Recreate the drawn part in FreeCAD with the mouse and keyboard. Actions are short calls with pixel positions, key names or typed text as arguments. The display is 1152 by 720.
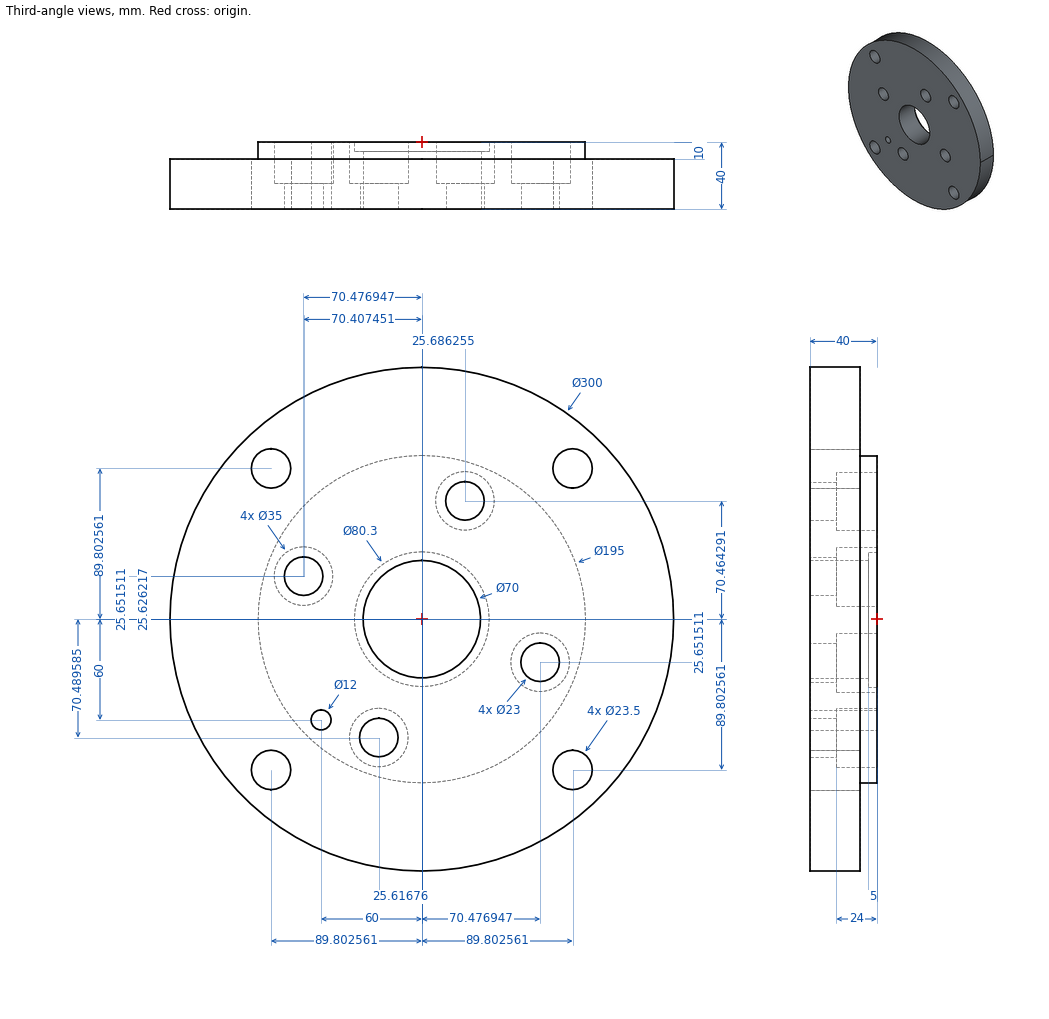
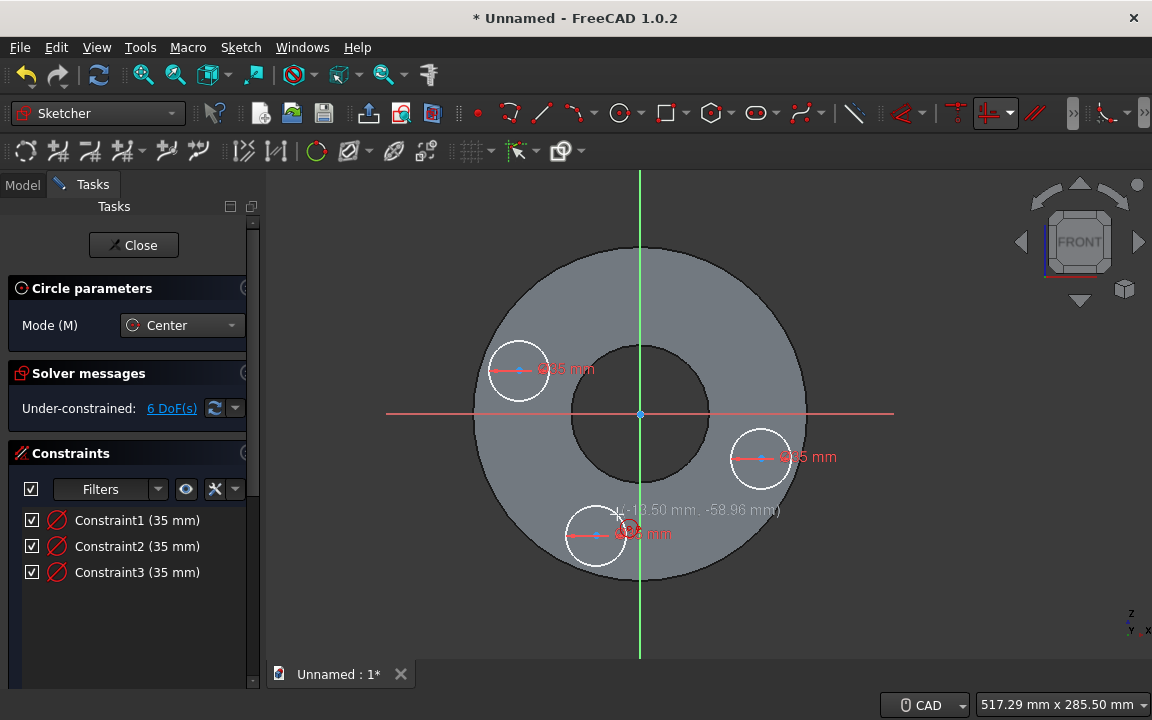
click(684, 293)
move(705, 272)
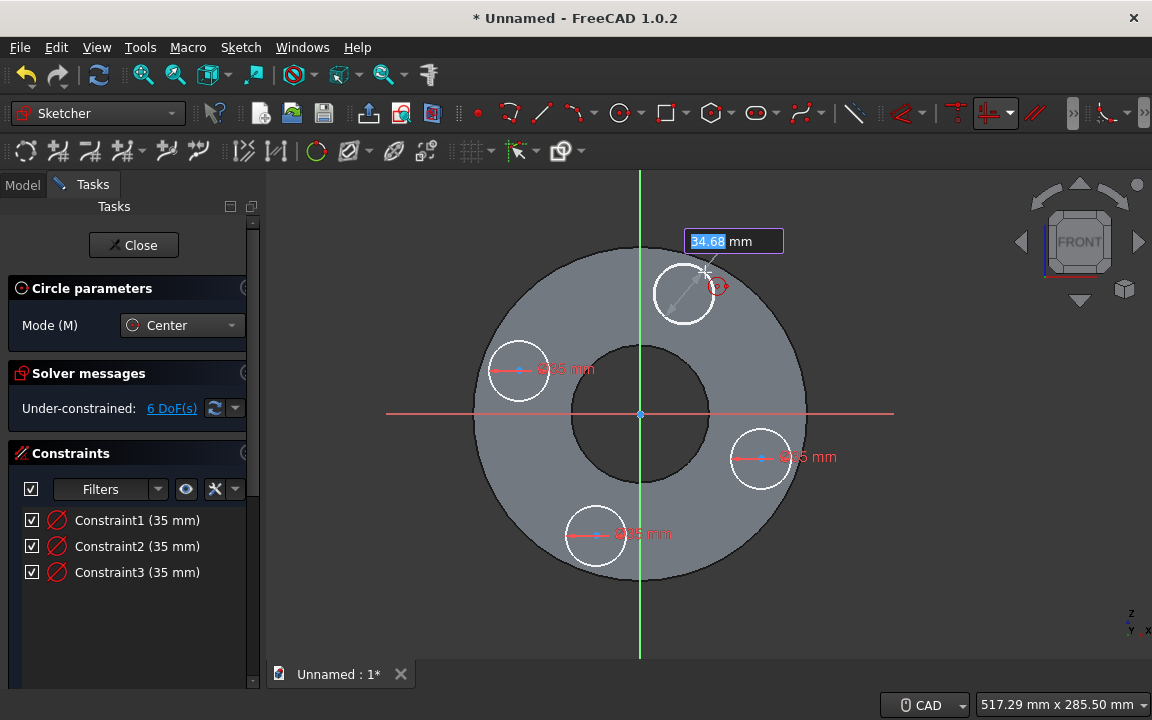
text(35)
key(Return)
key(Escape)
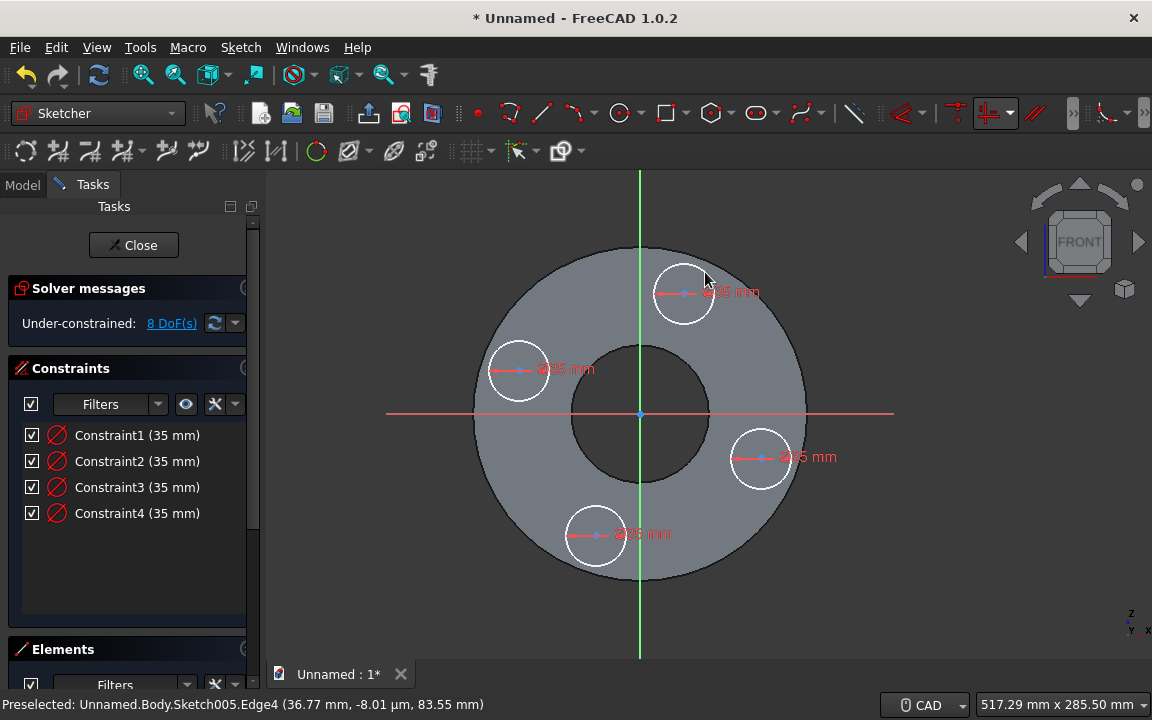
click(902, 114)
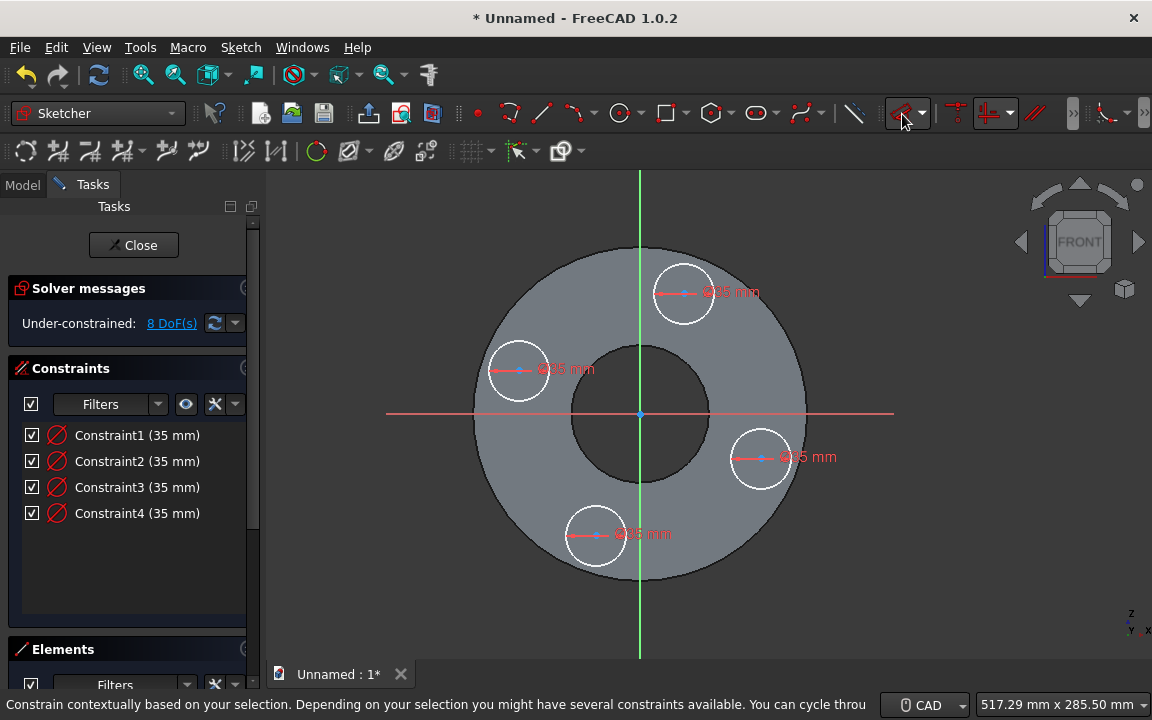
click(596, 536)
click(618, 380)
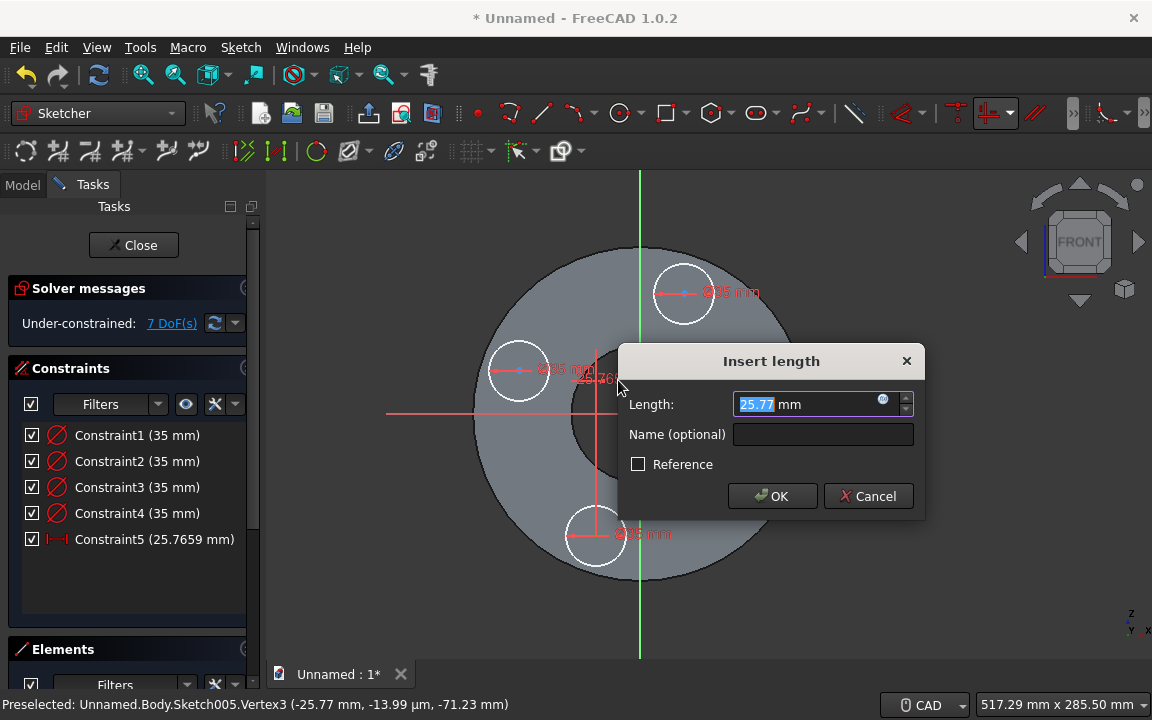
text(25.61676)
key(Return)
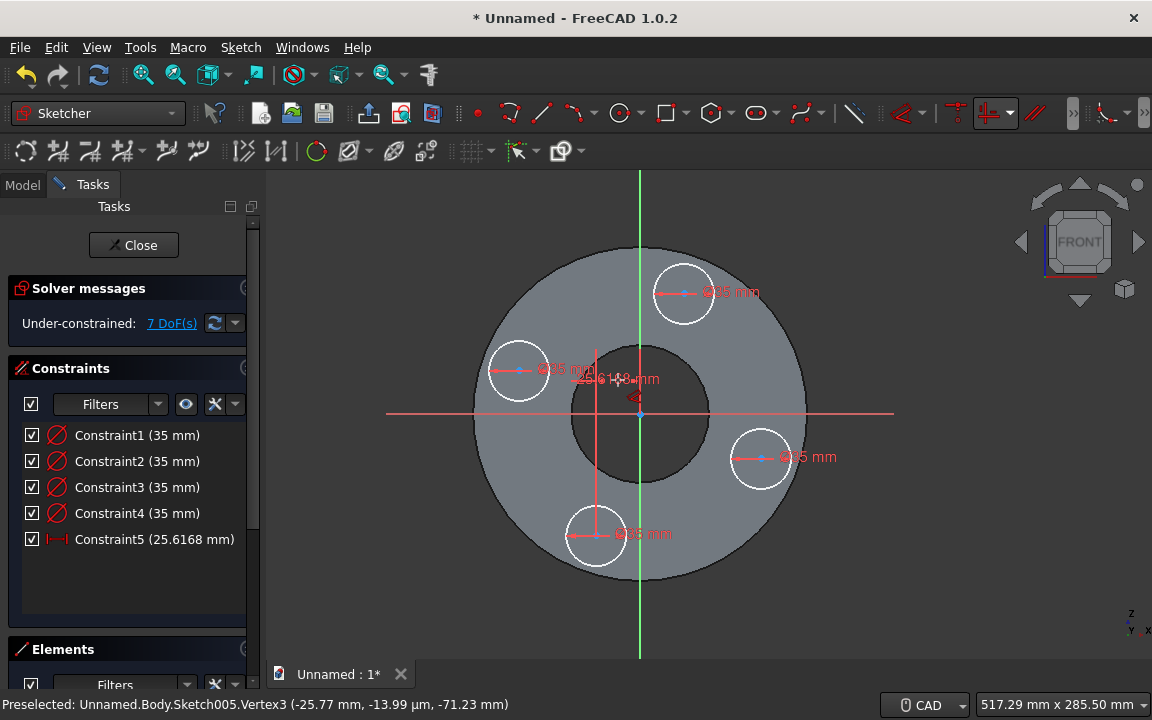
click(519, 371)
click(580, 337)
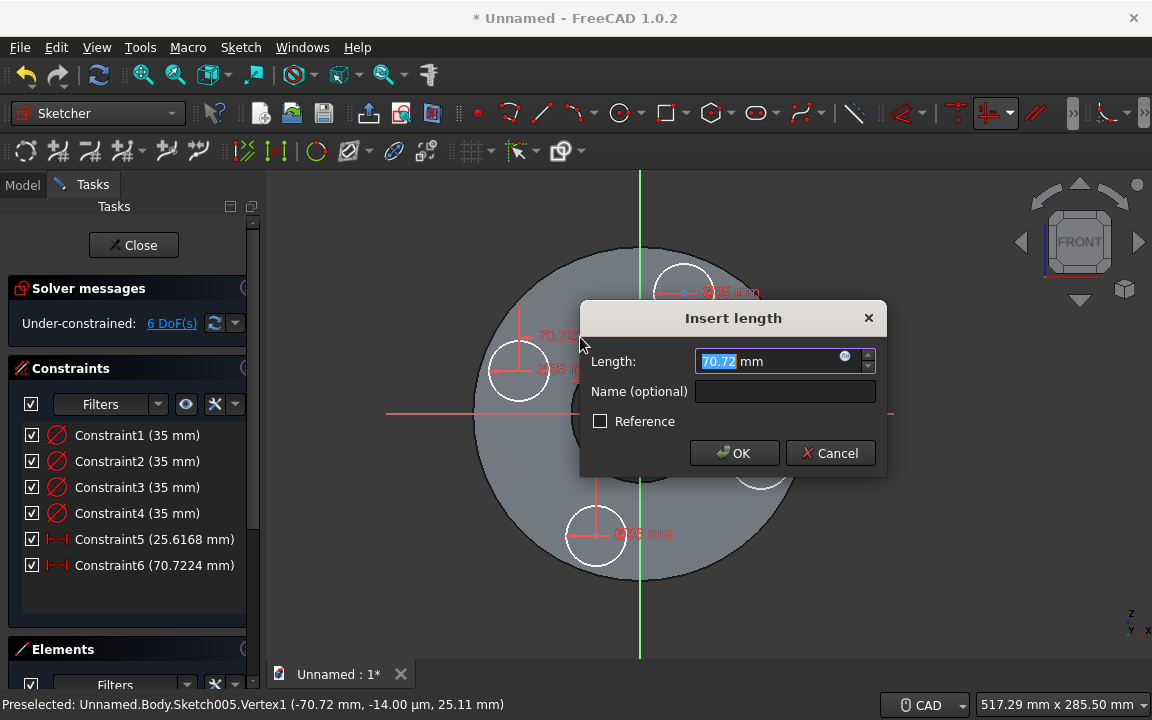
text(70.476947)
key(Return)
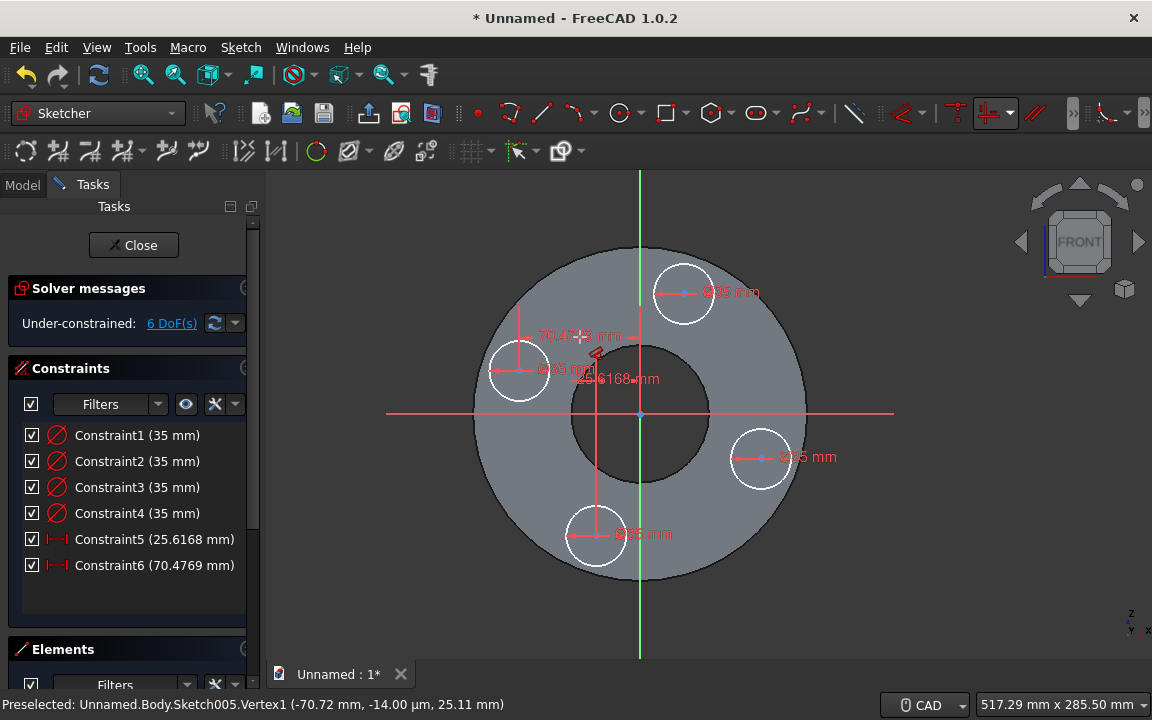
click(519, 371)
click(461, 393)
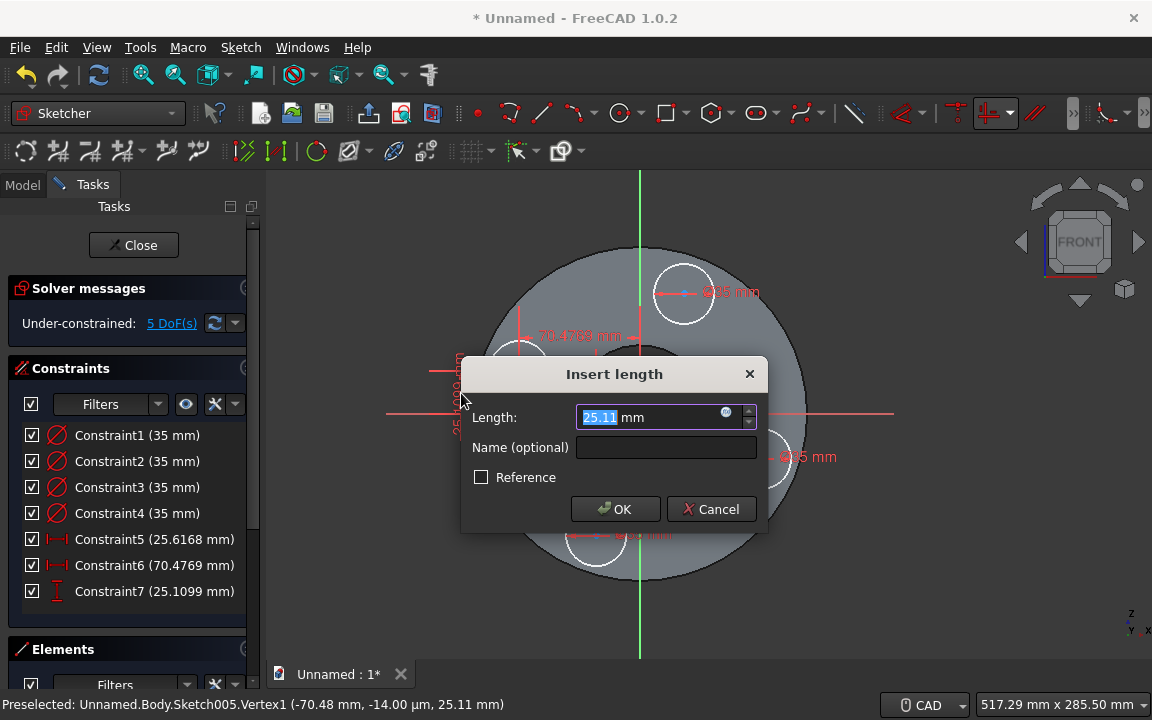
text(25.651511)
key(Return)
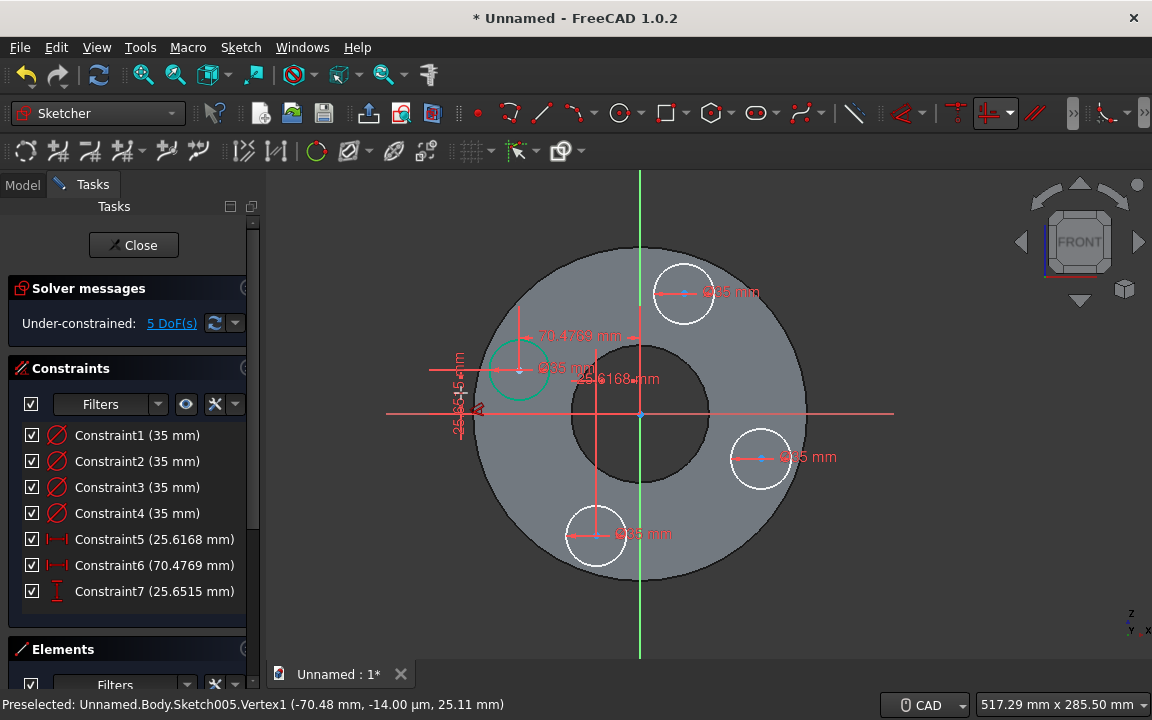
click(761, 459)
click(701, 493)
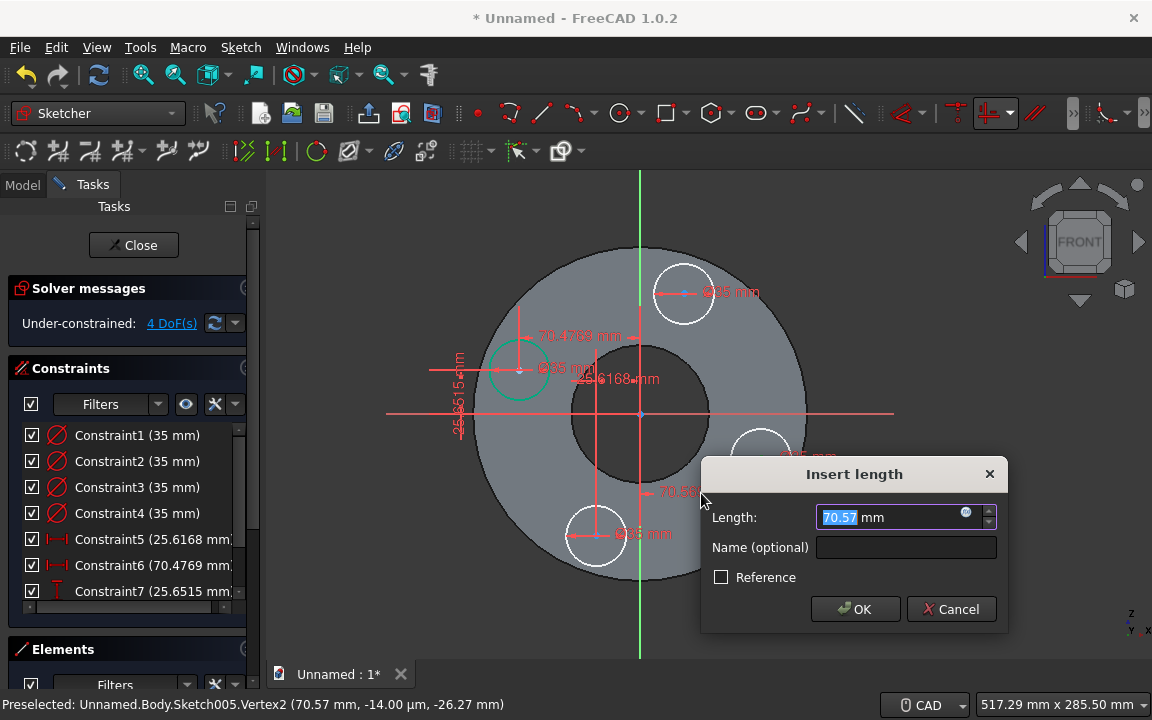
text(70.476947)
key(Return)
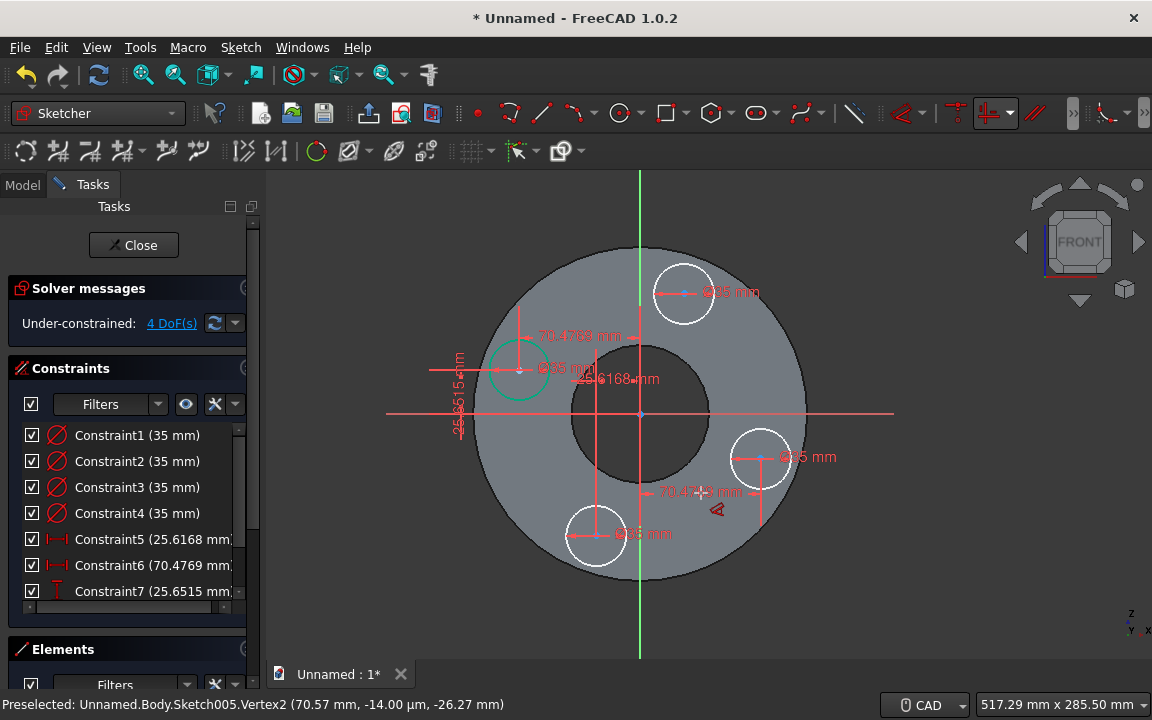
click(761, 459)
click(606, 437)